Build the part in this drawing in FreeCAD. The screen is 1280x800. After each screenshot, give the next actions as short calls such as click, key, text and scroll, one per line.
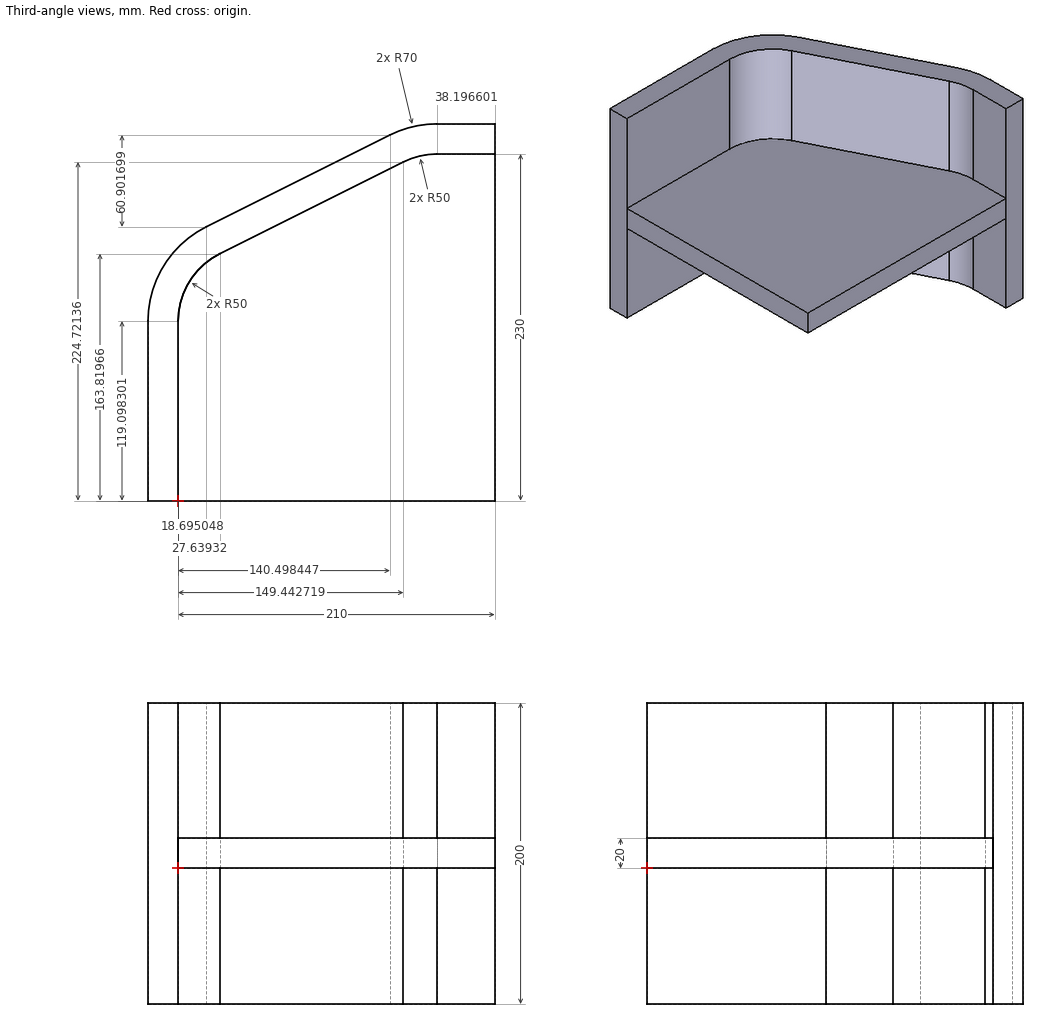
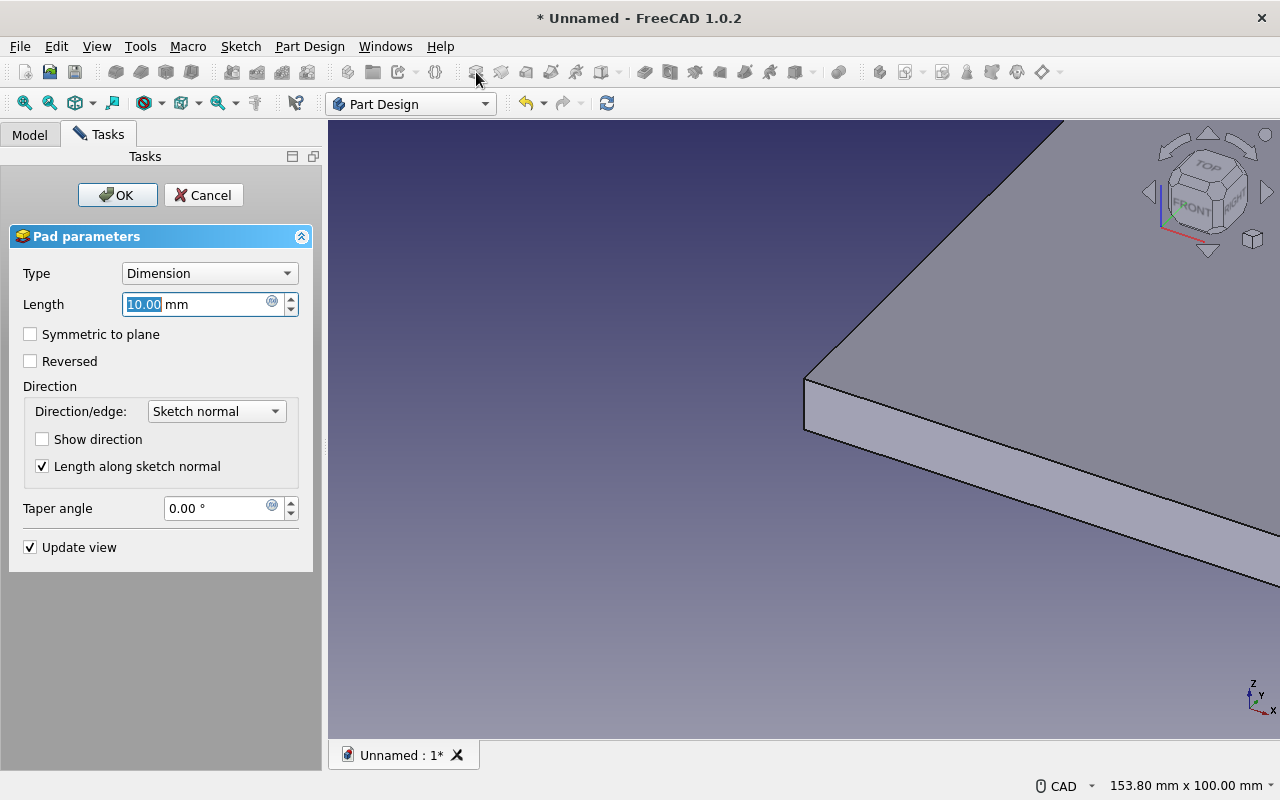
text(20)
key(Tab)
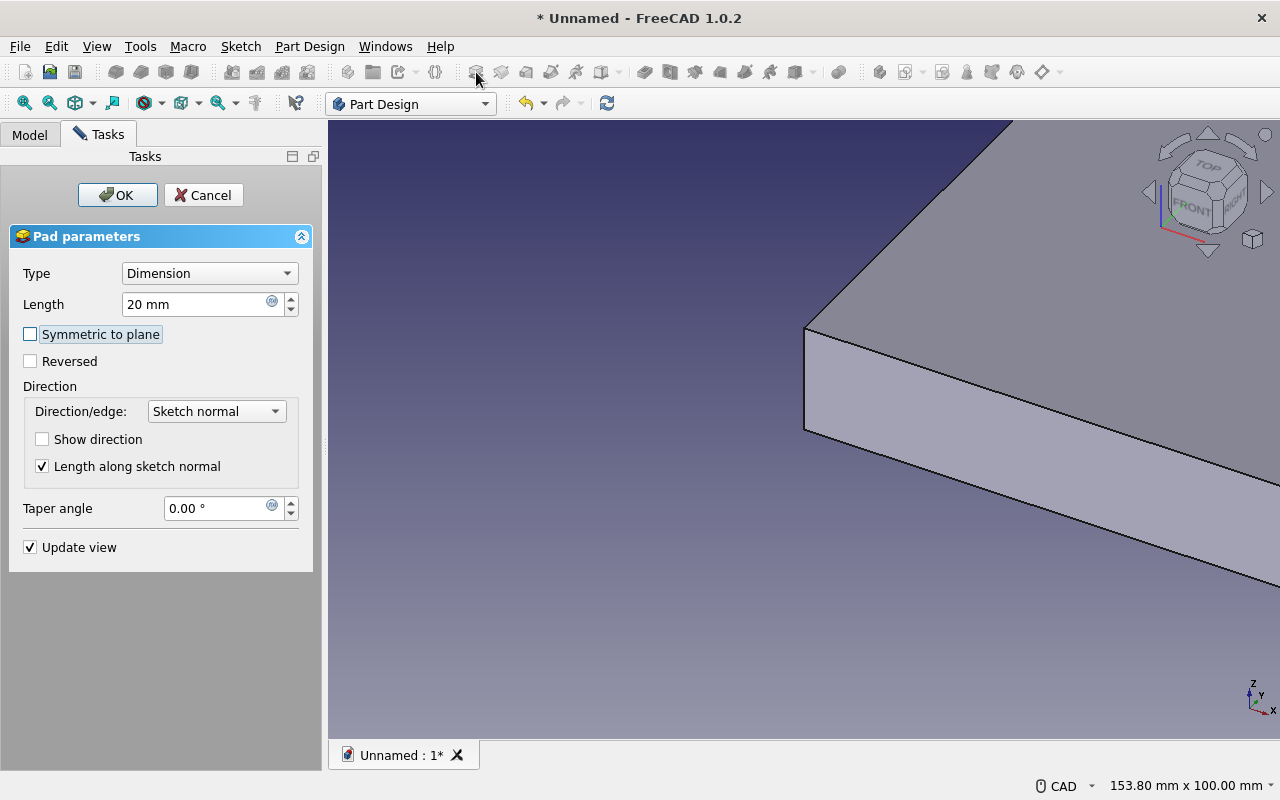
click(118, 195)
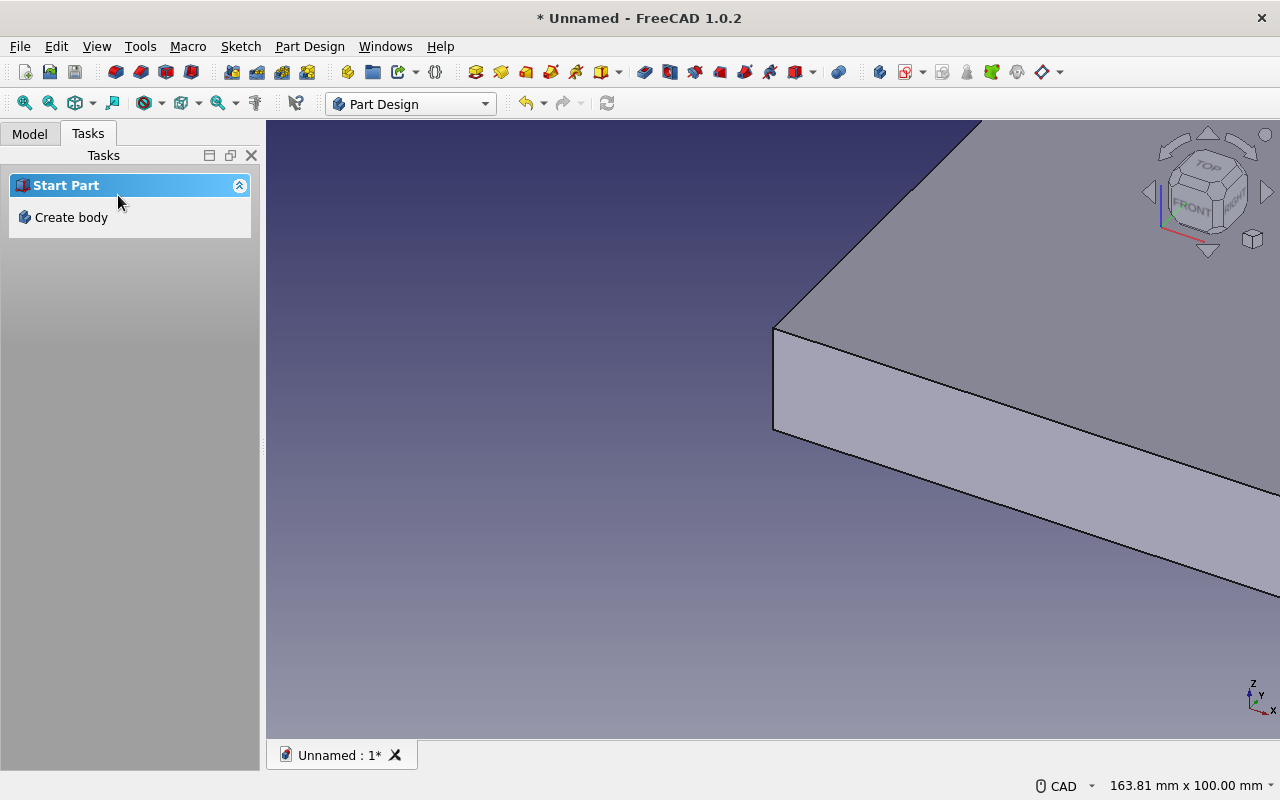
click(25, 104)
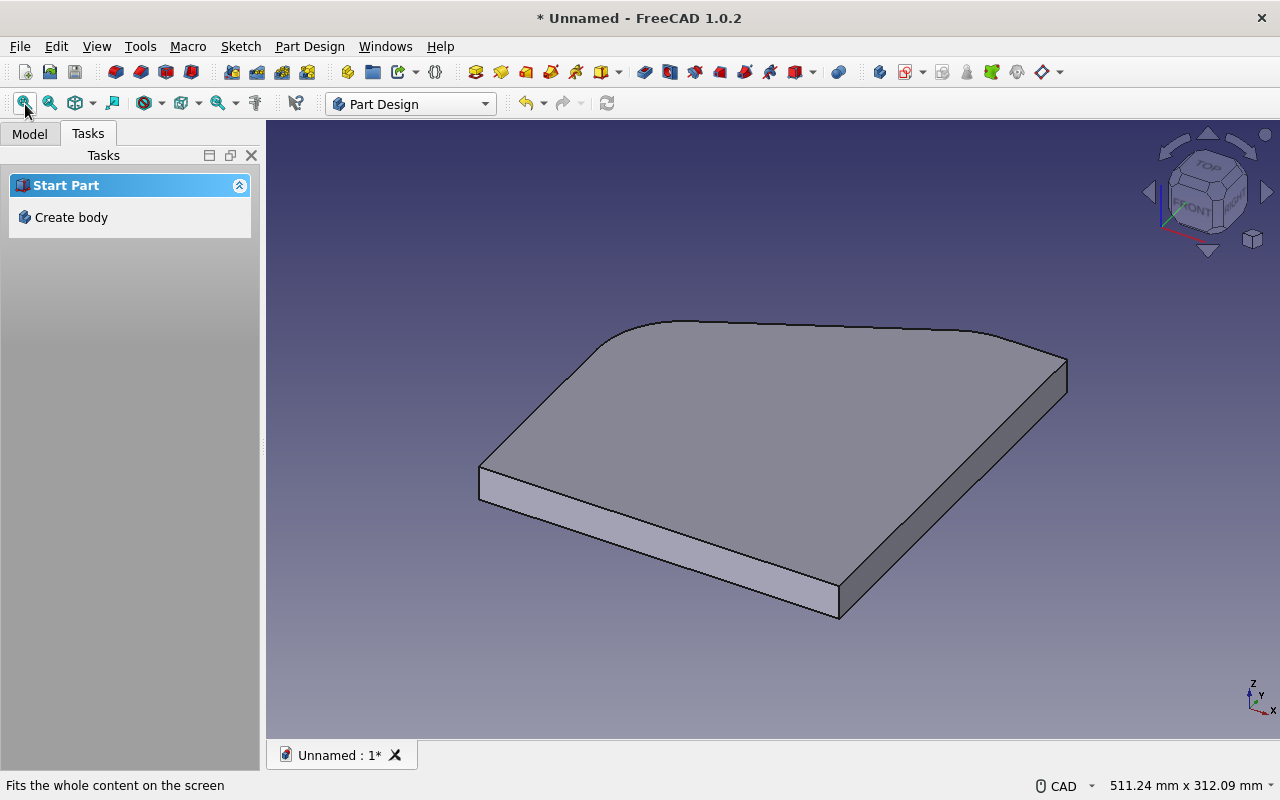
click(880, 72)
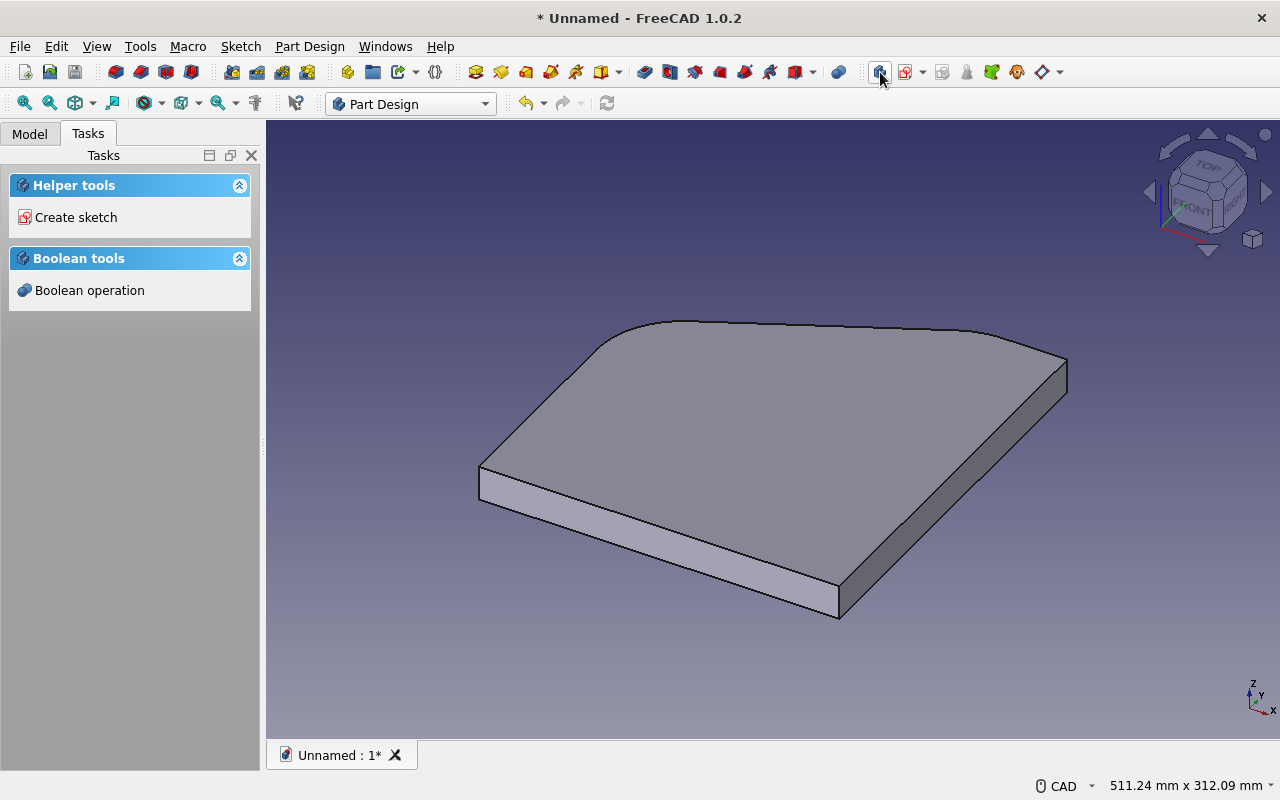
click(30, 134)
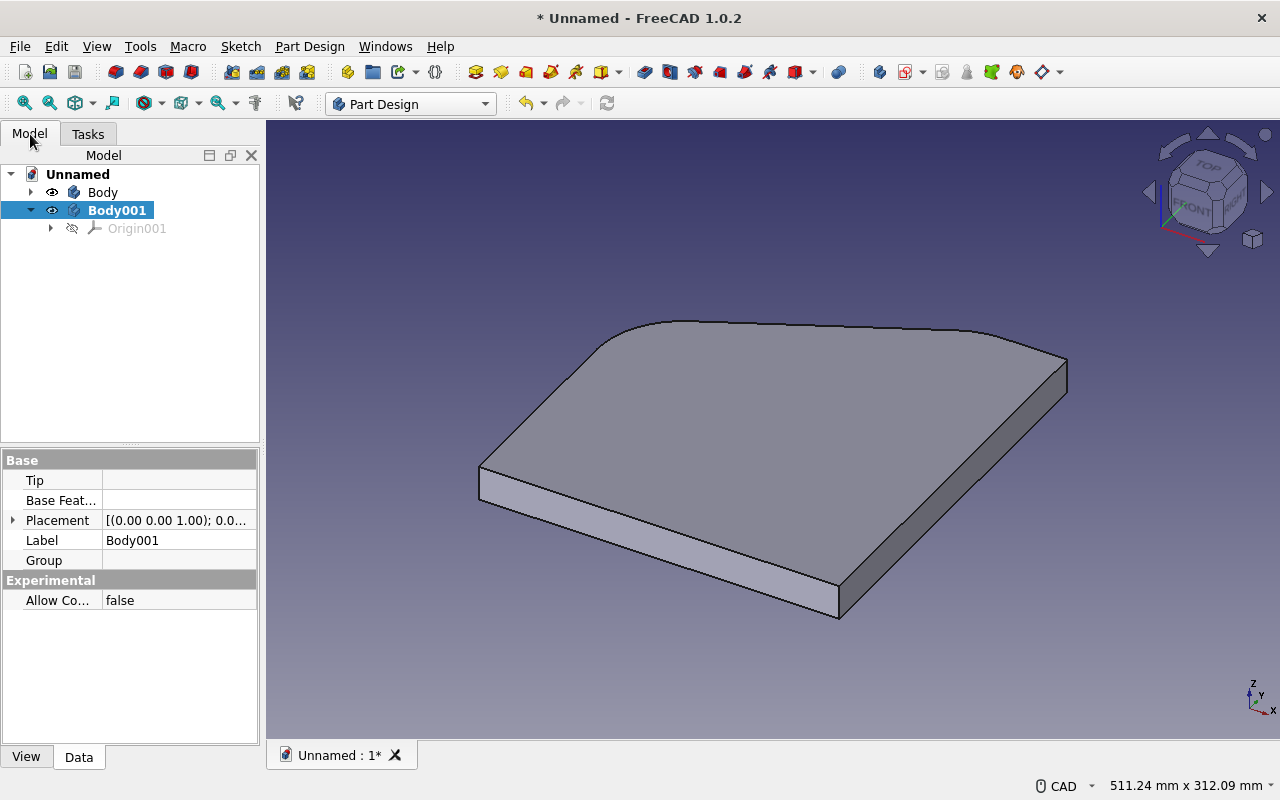
click(51, 228)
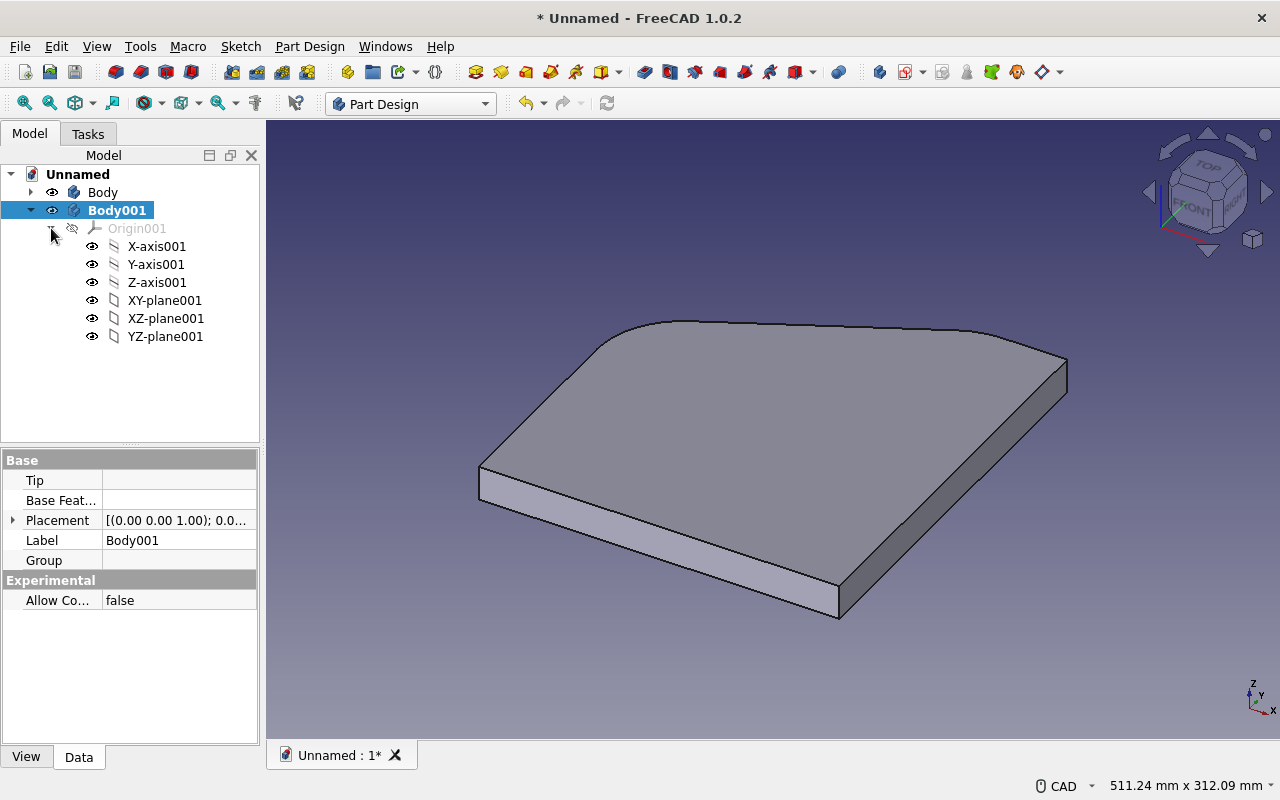
click(137, 300)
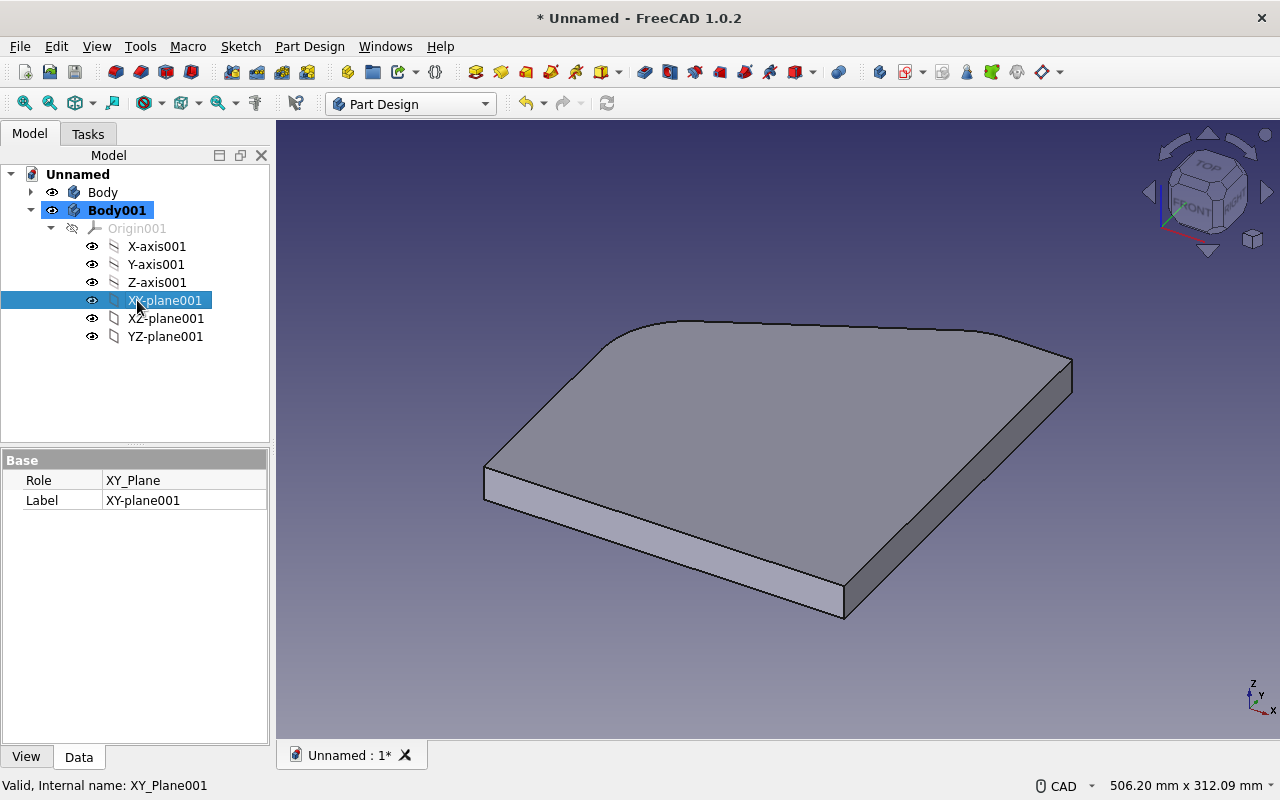
click(1042, 72)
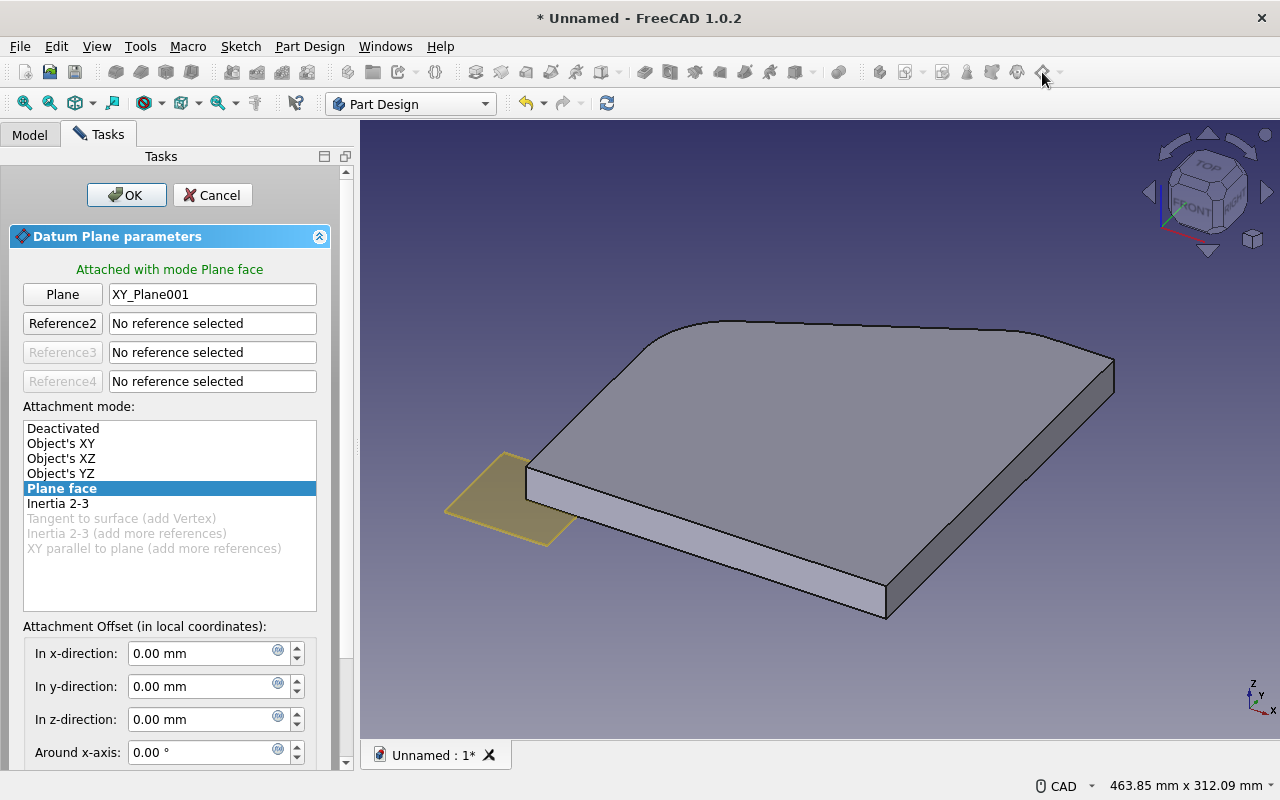
triple_click(210, 720)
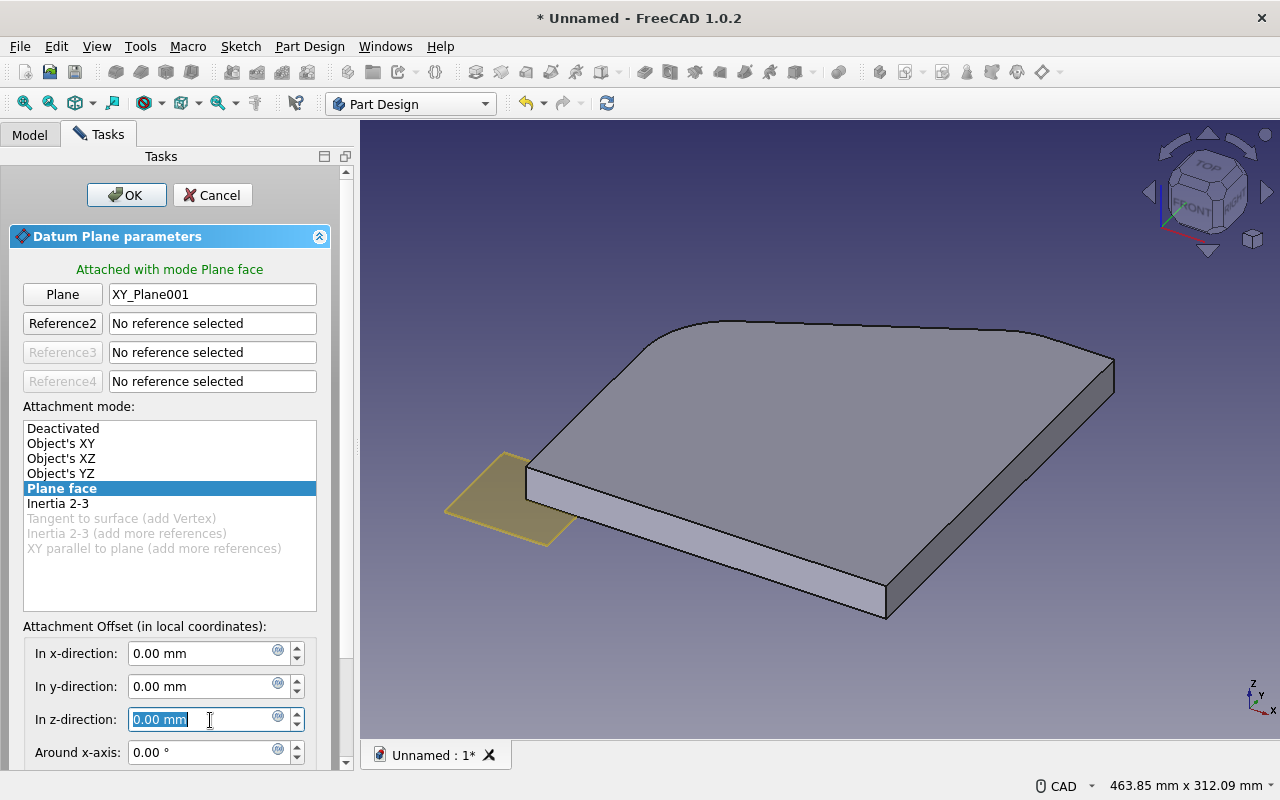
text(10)
key(Tab)